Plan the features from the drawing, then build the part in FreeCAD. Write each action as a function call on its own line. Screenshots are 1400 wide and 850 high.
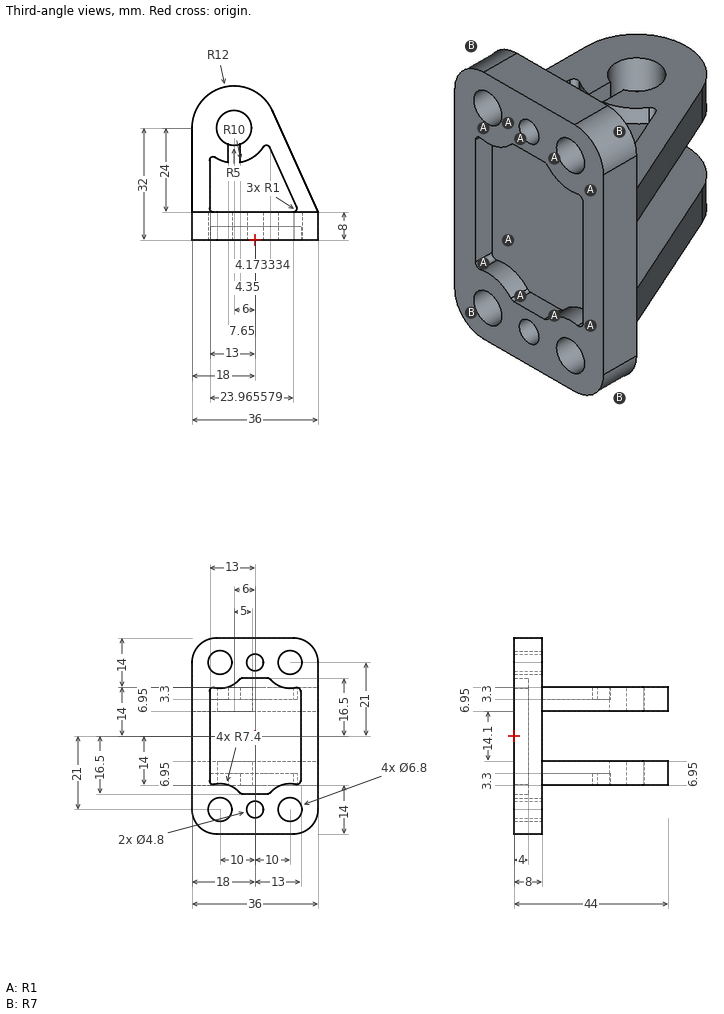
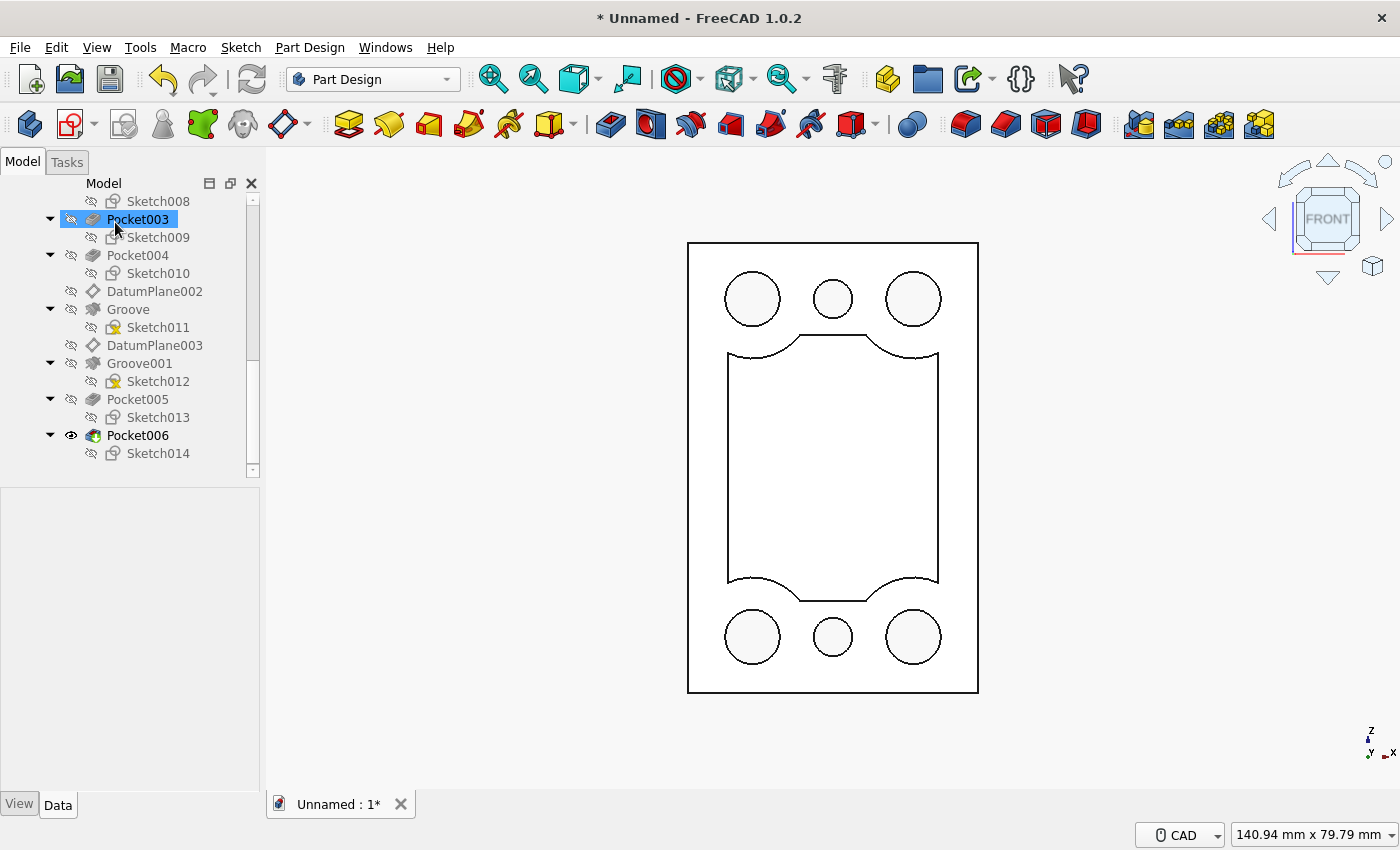
key(3)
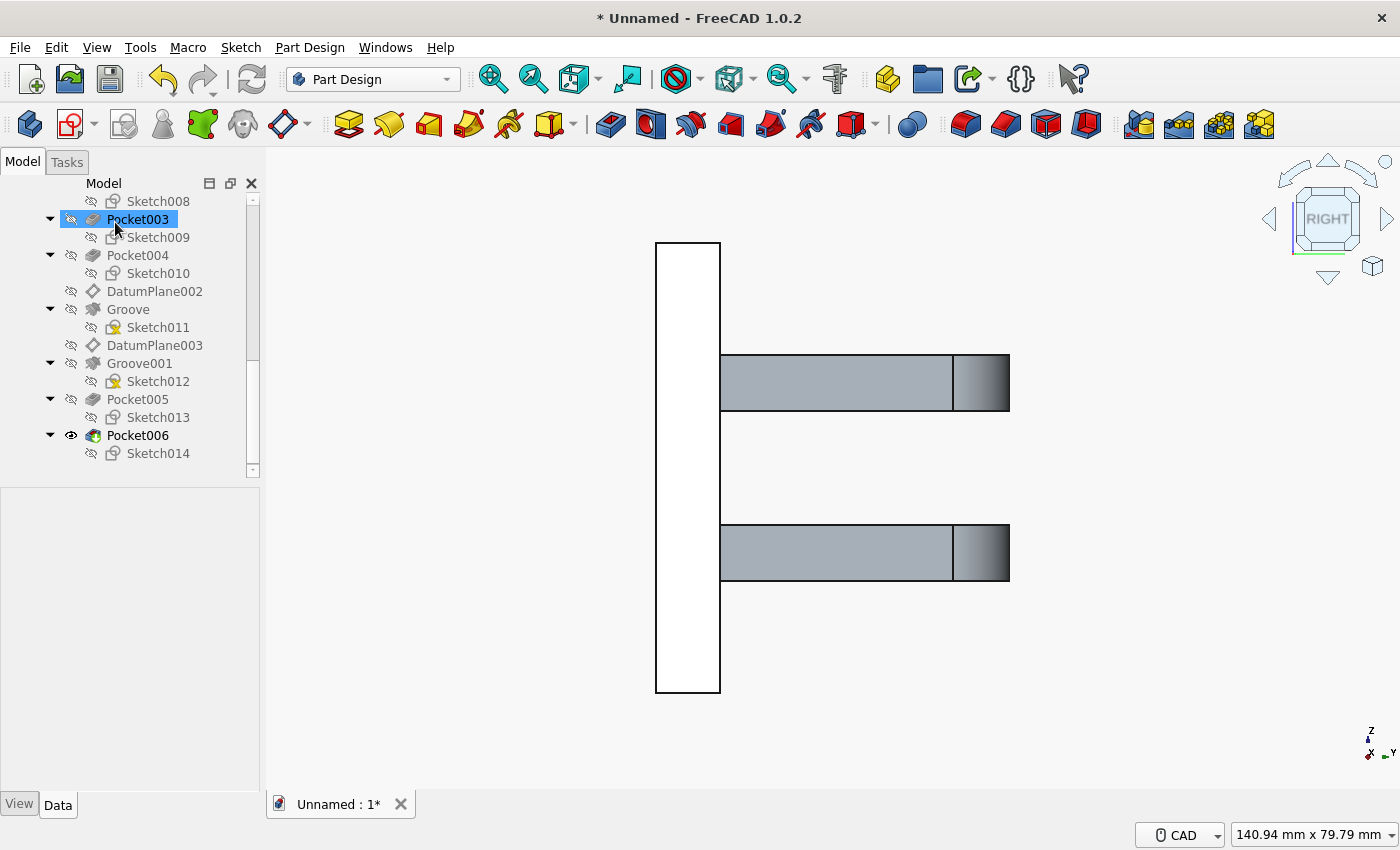
key(5)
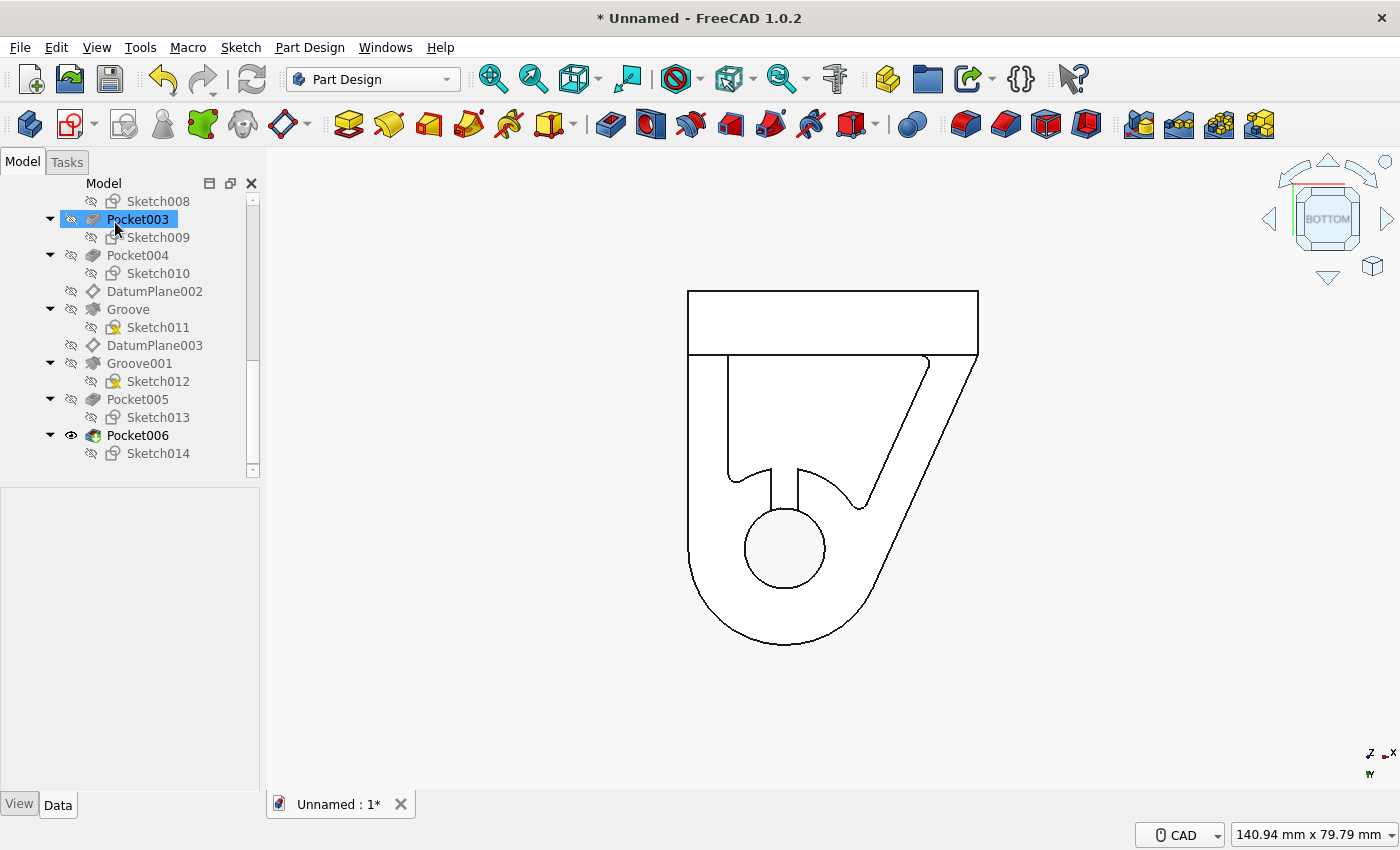
key(4)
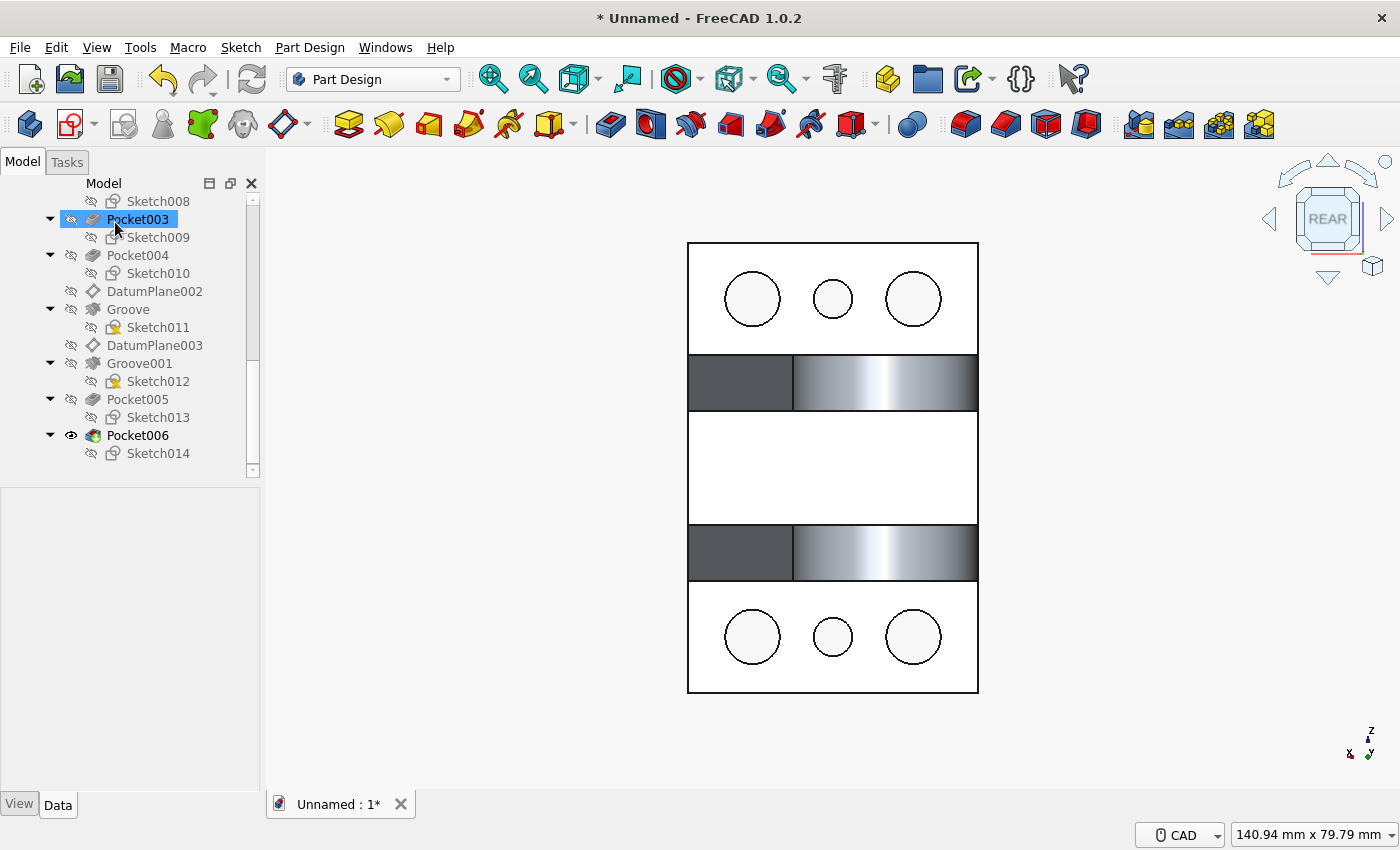
key(6)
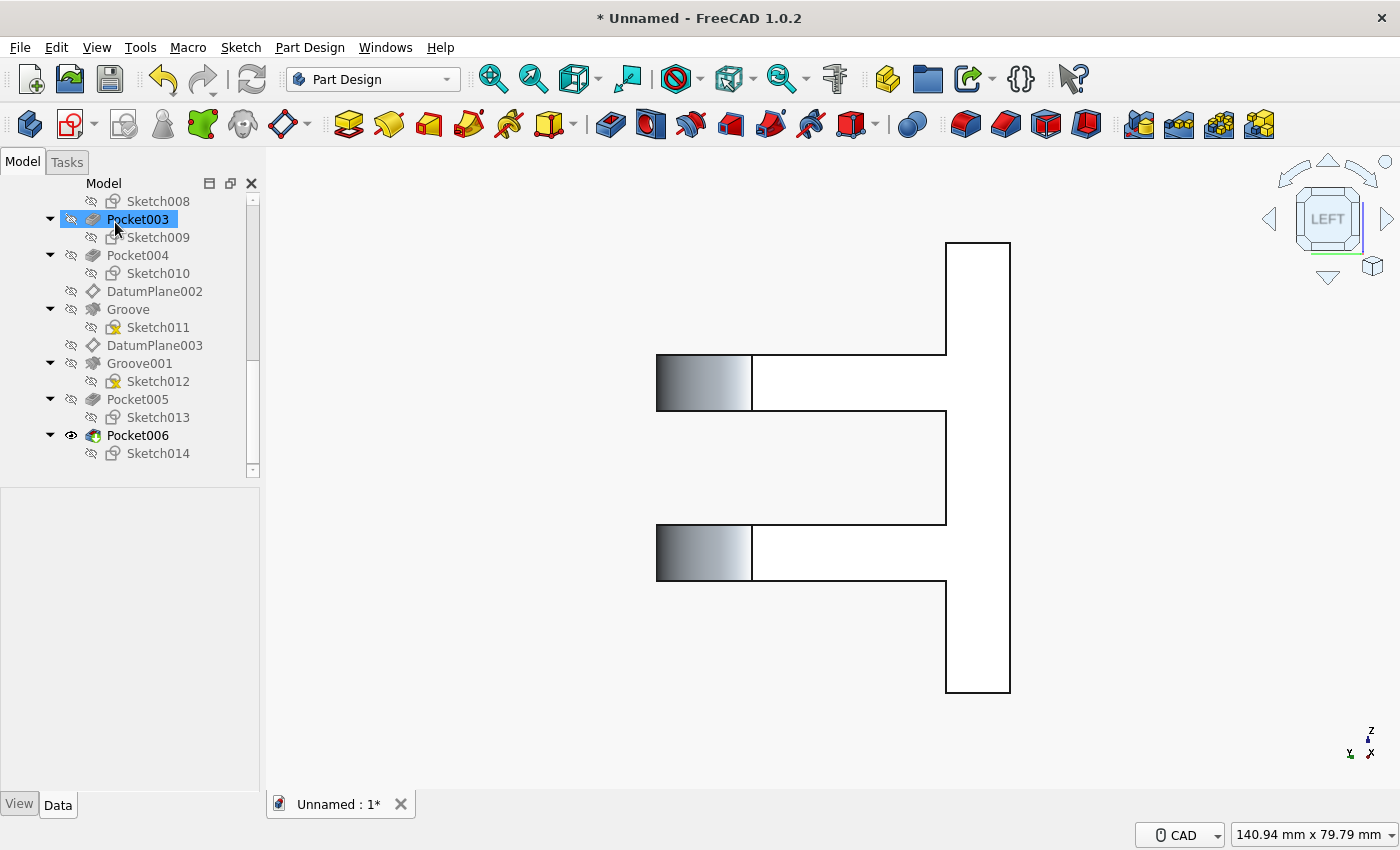
key(v)
key(3)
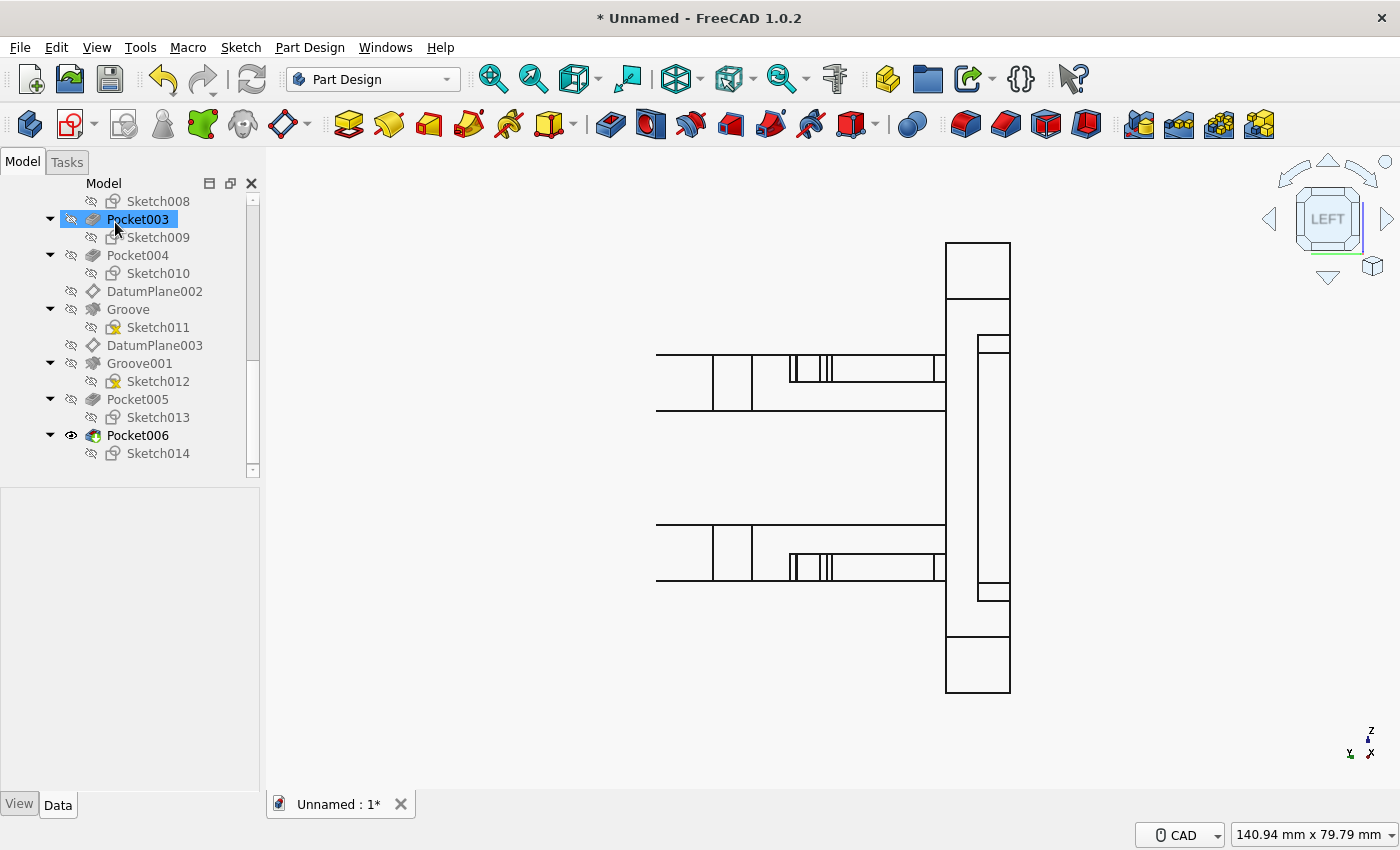
key(0)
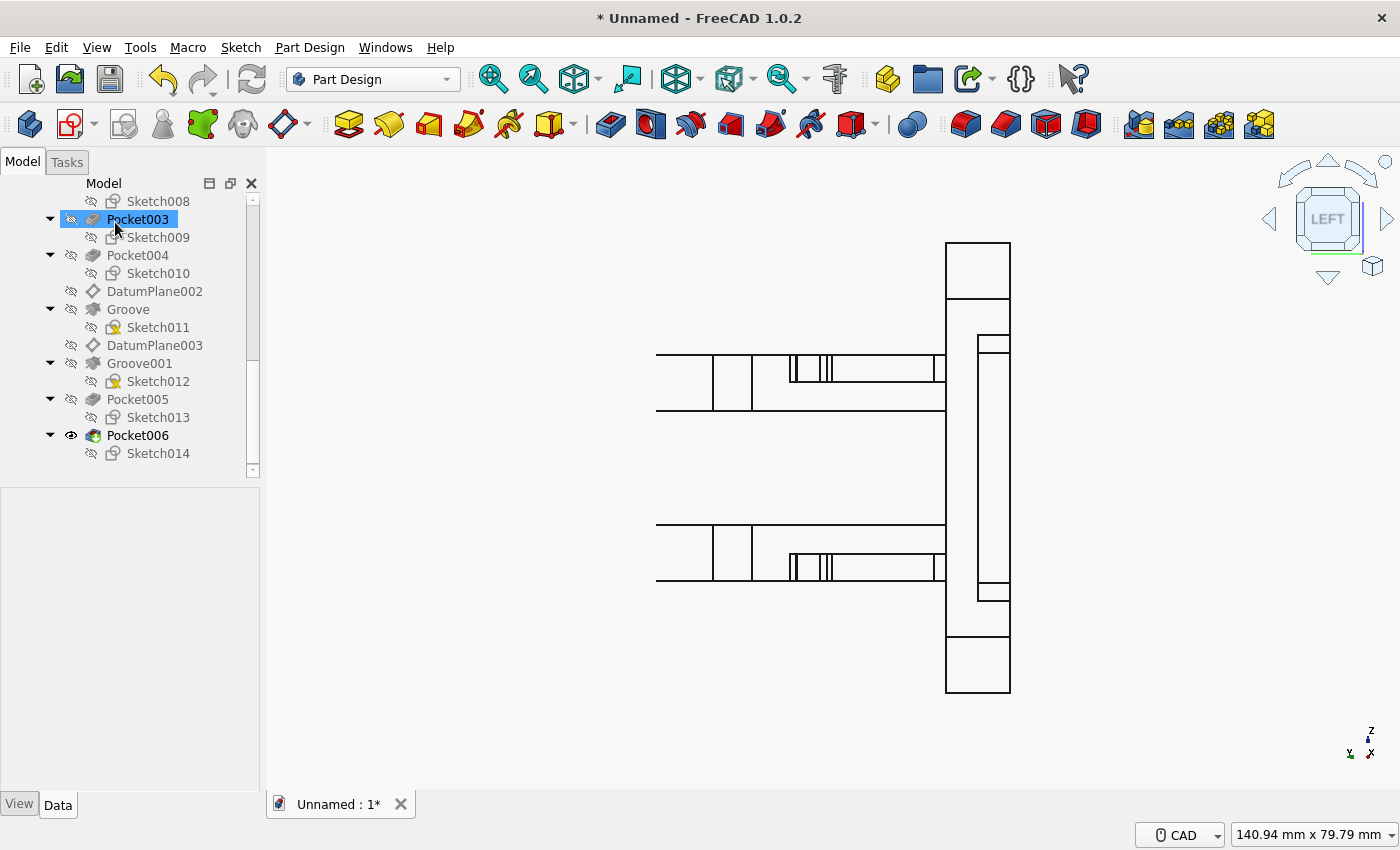
click(679, 551)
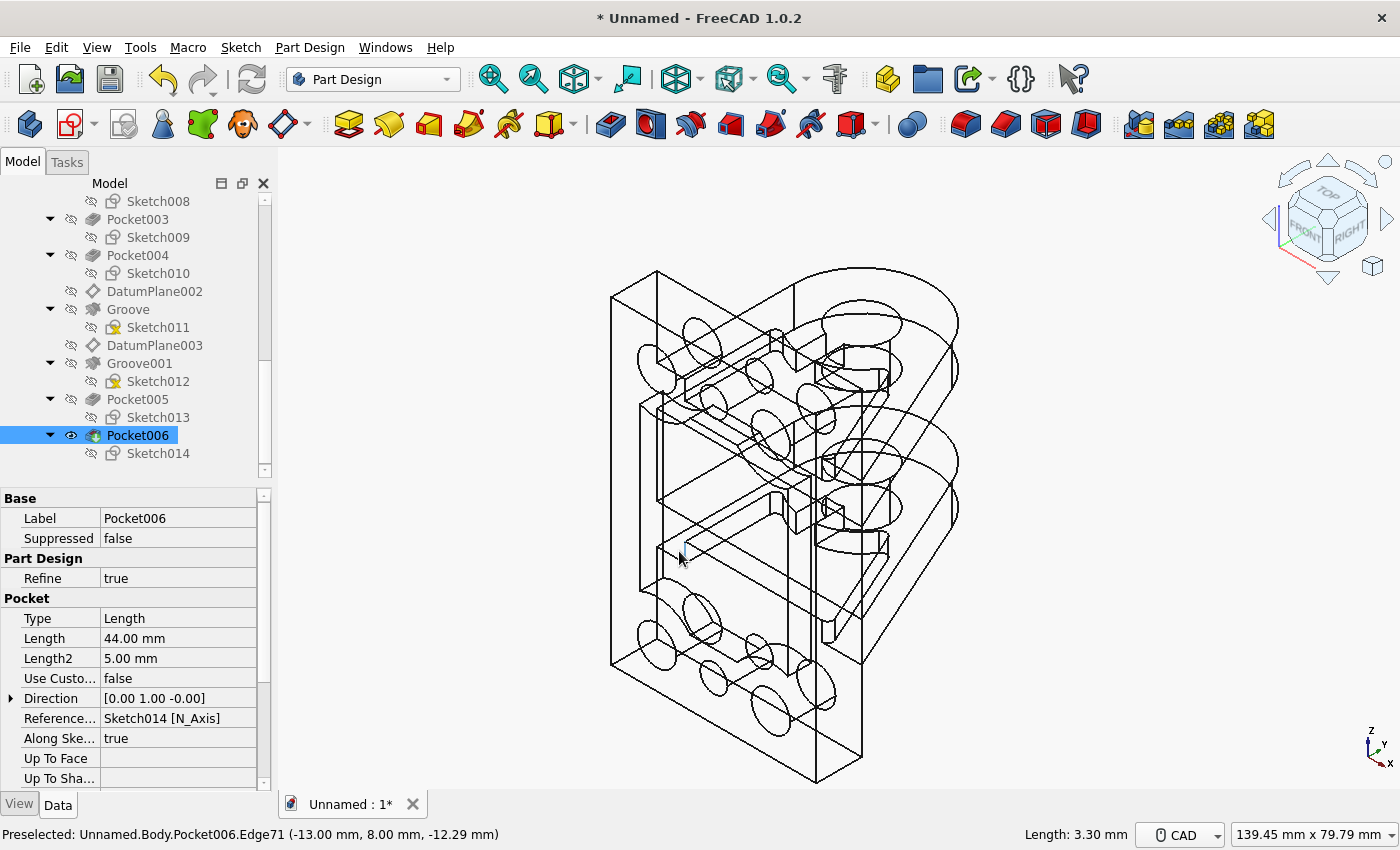
click(651, 396, ctrl)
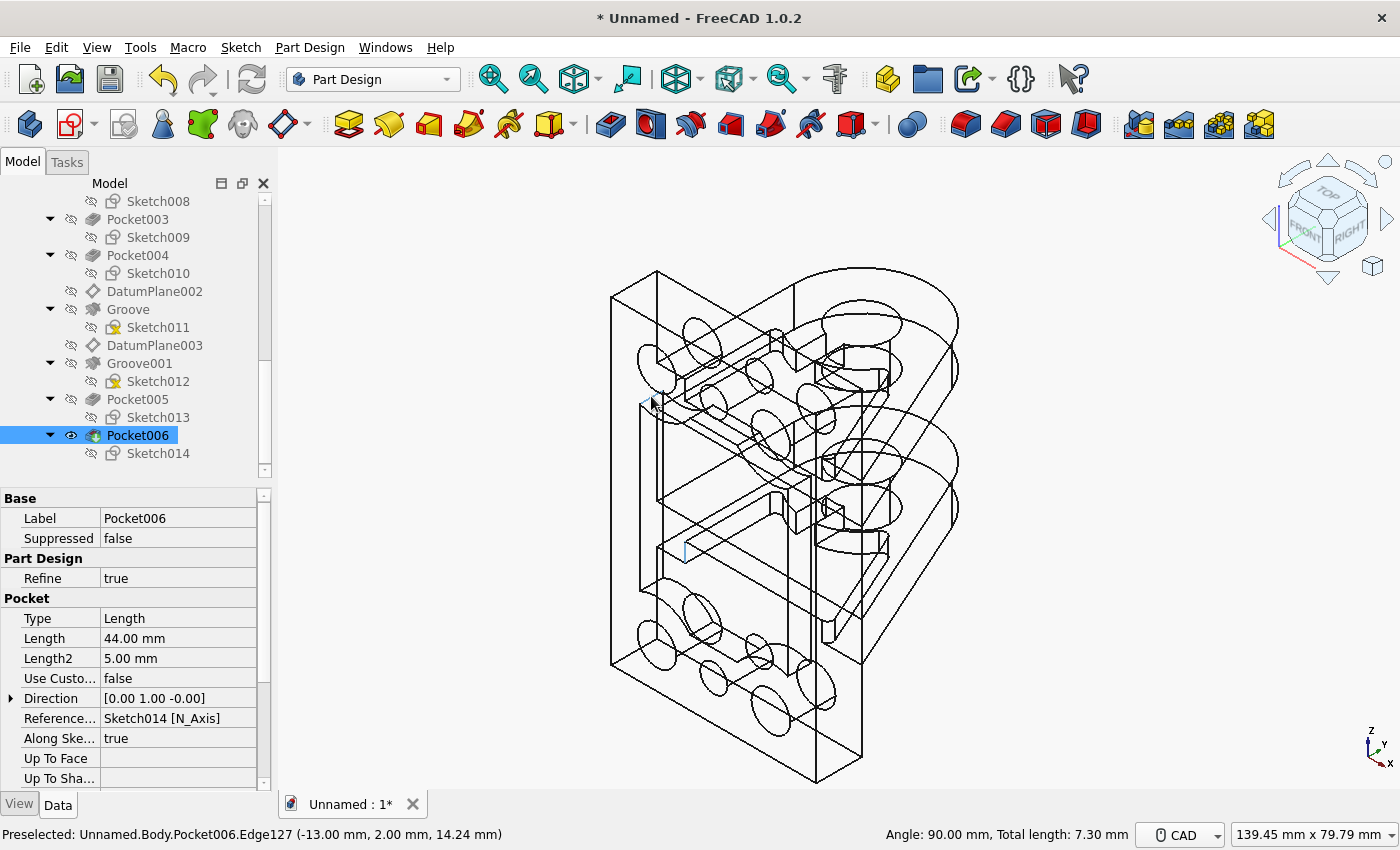
click(697, 413, ctrl)